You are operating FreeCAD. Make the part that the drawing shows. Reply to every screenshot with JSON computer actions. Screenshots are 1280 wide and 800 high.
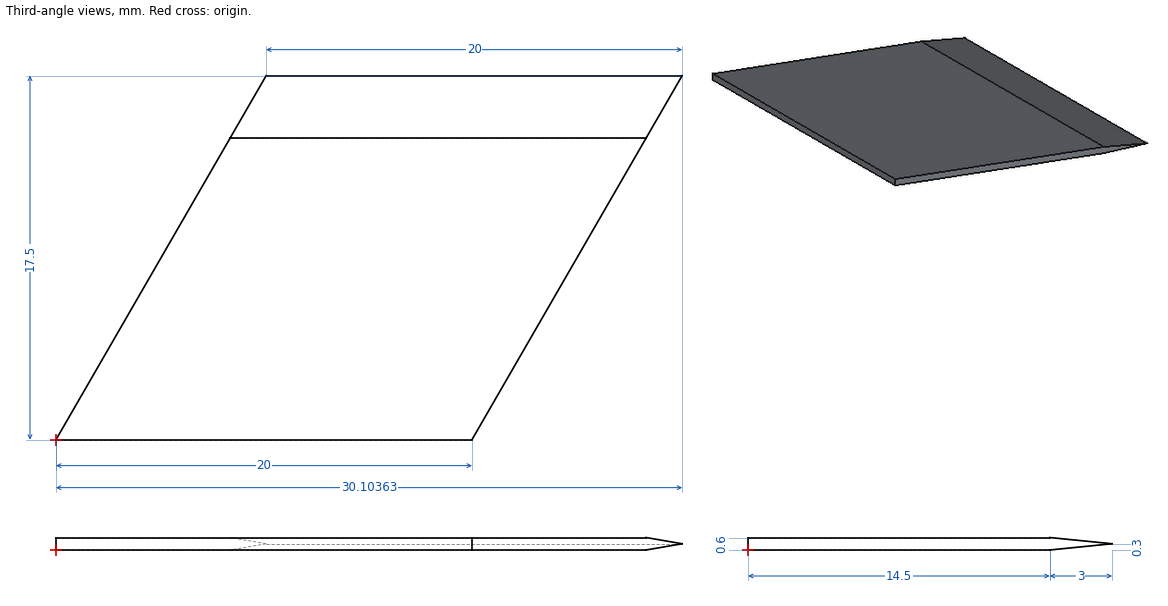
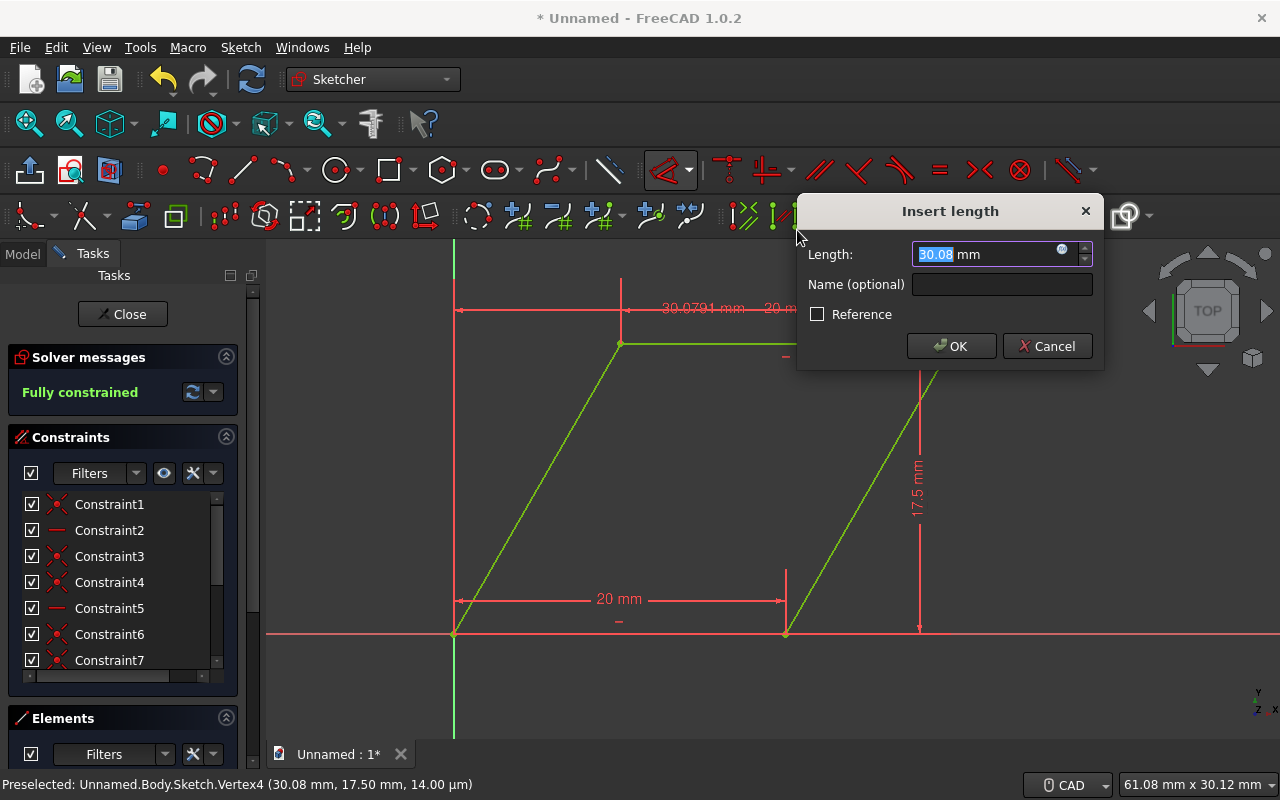
{"action": "type", "text": "30.10363"}
{"action": "key", "text": "Return"}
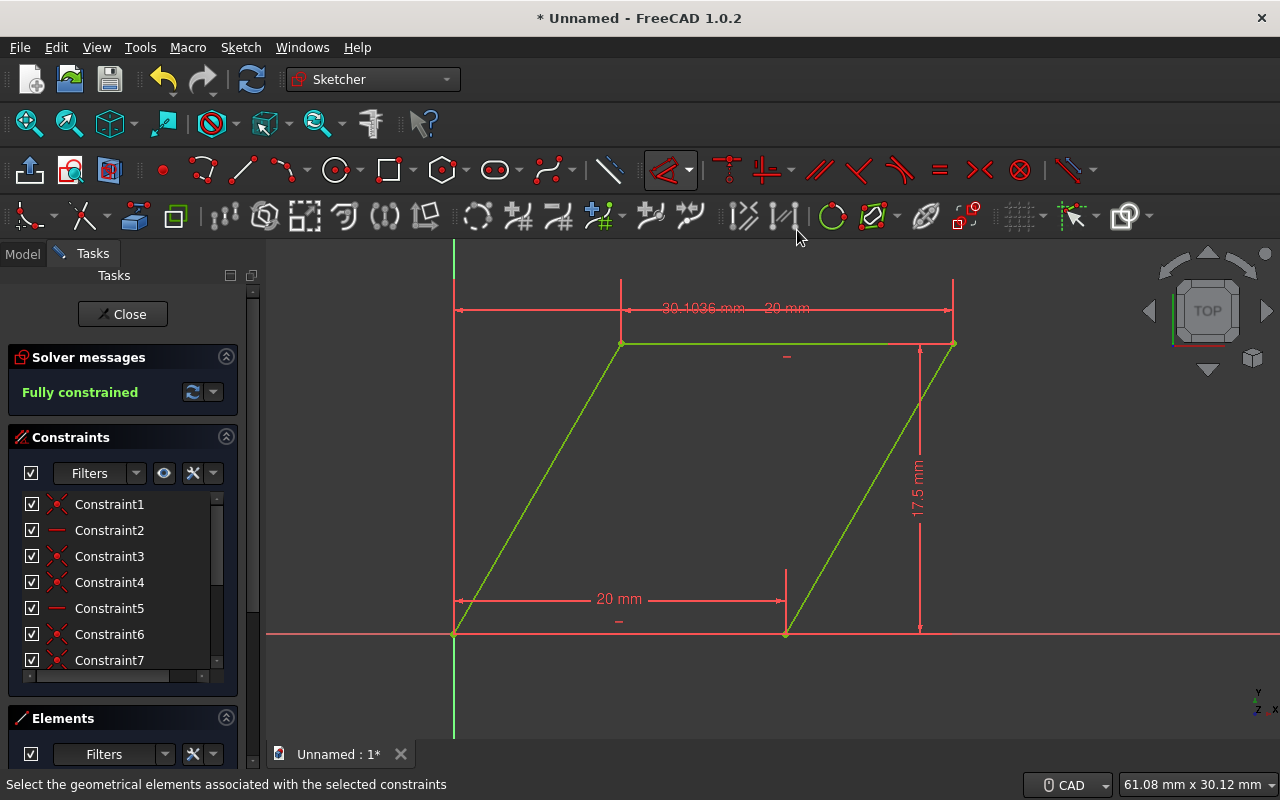
{"action": "left_click", "coordinate": [123, 314]}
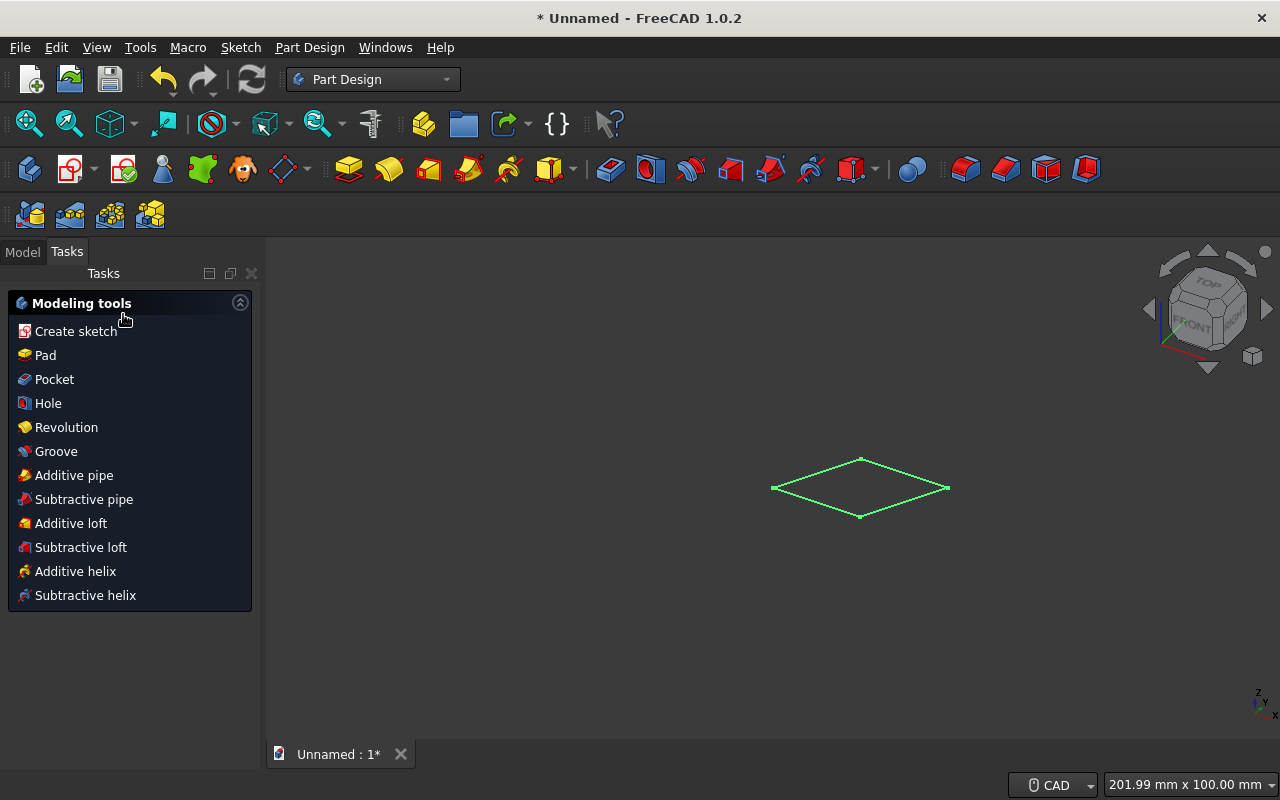
{"action": "left_click", "coordinate": [350, 170]}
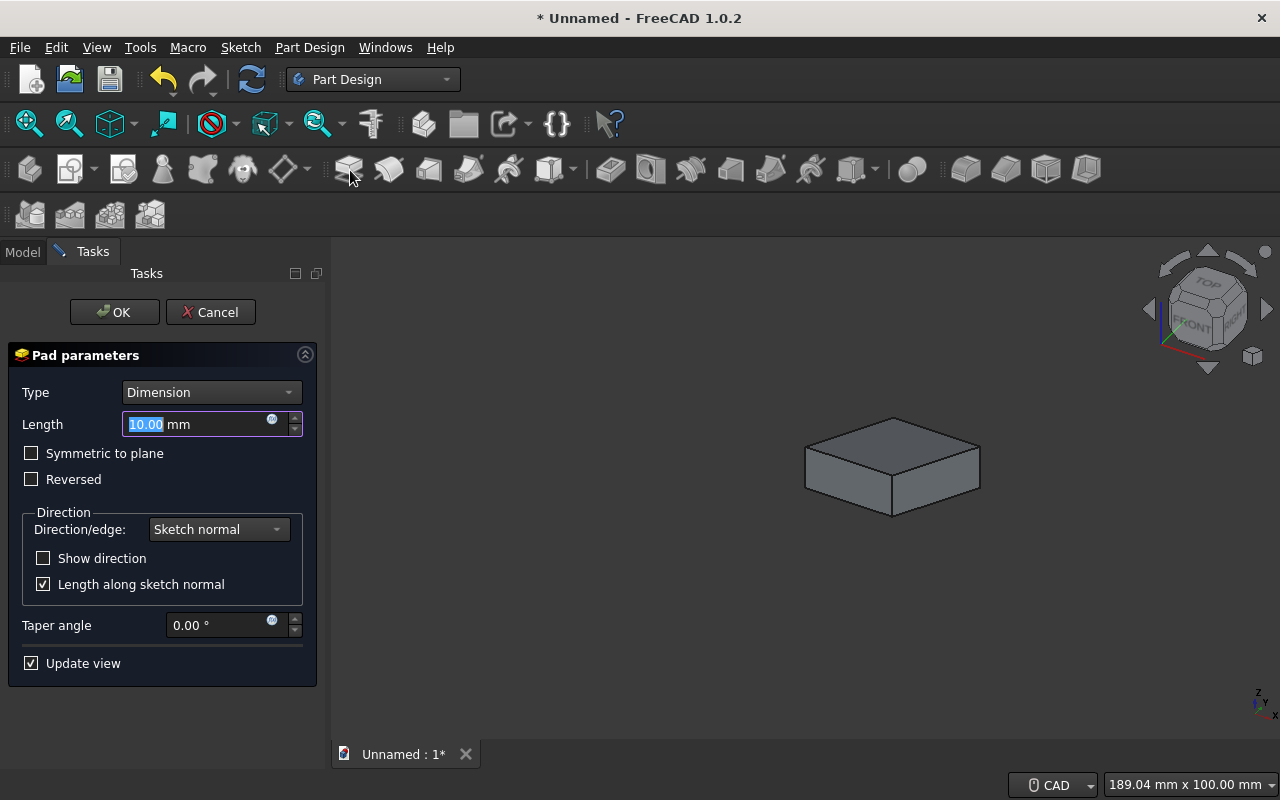
{"action": "type", "text": "0.6"}
{"action": "key", "text": "Tab"}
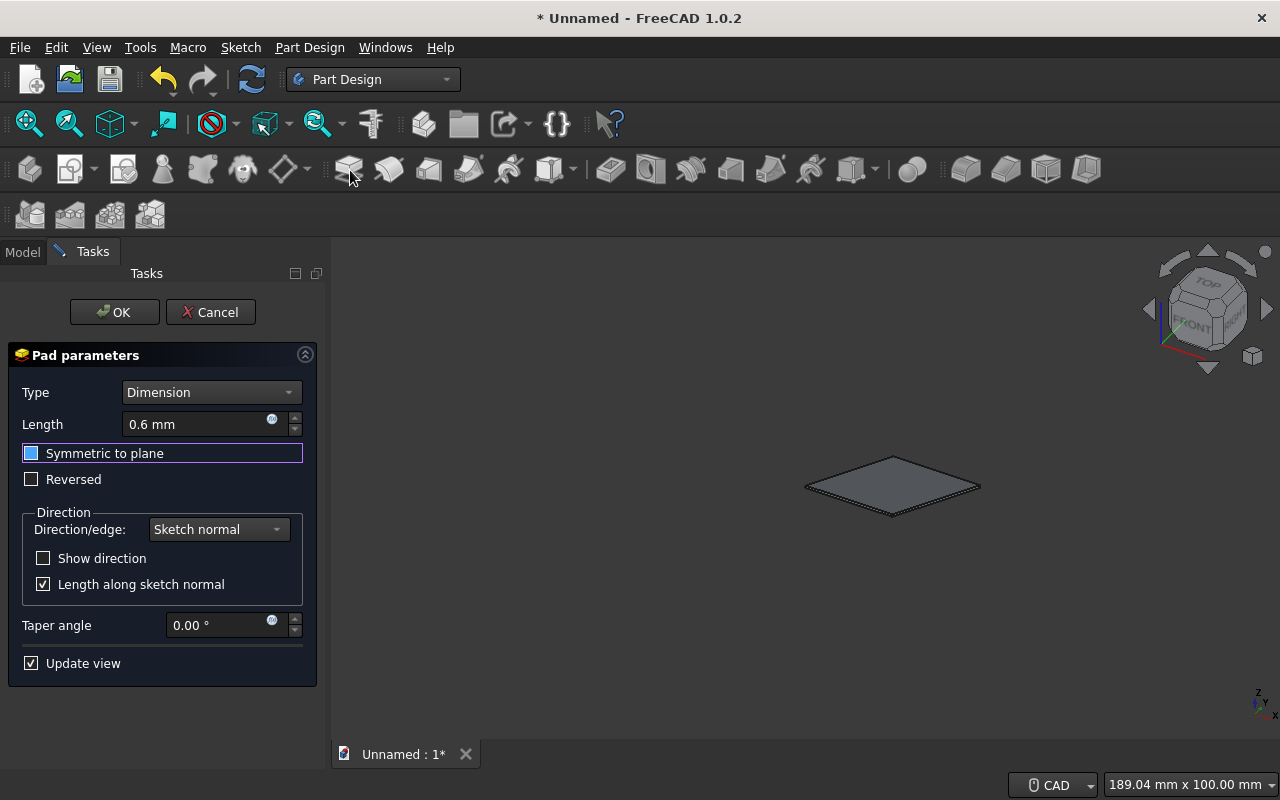
{"action": "left_click", "coordinate": [115, 312]}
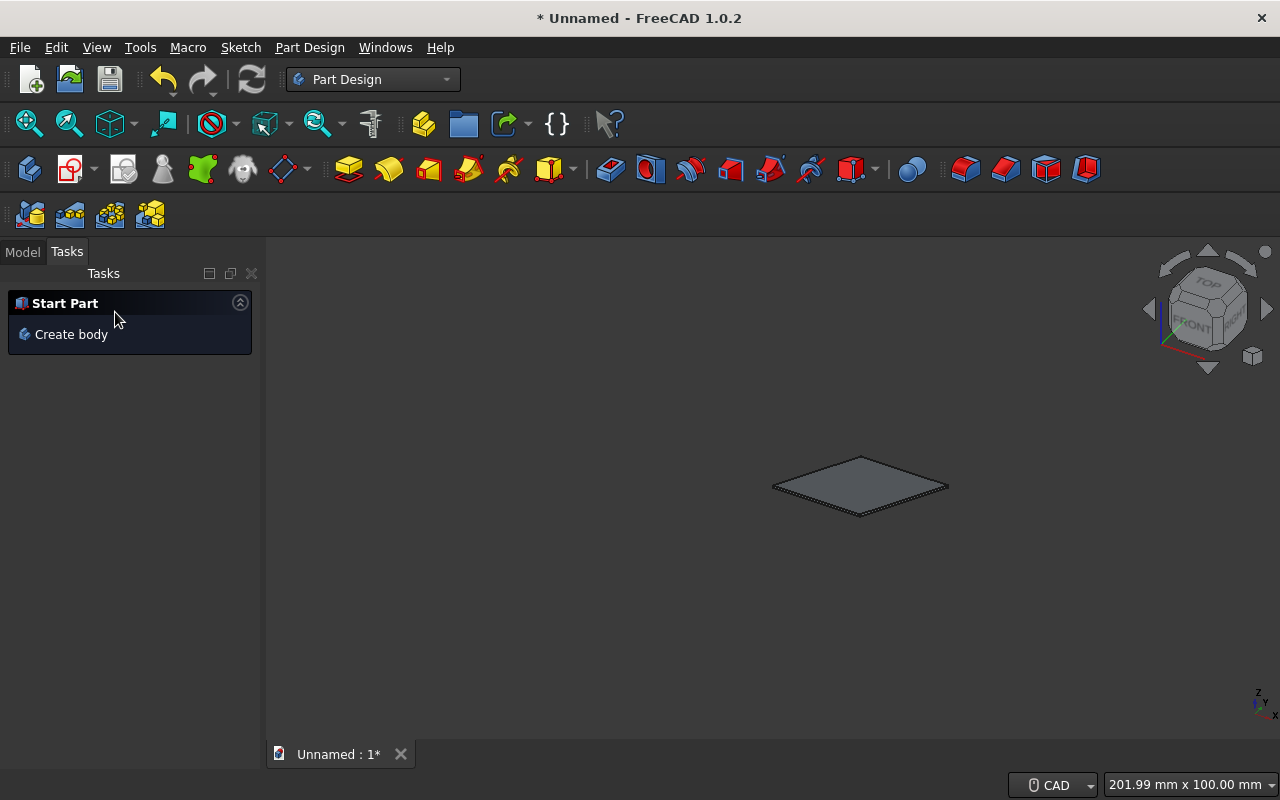
{"action": "left_click", "coordinate": [30, 124]}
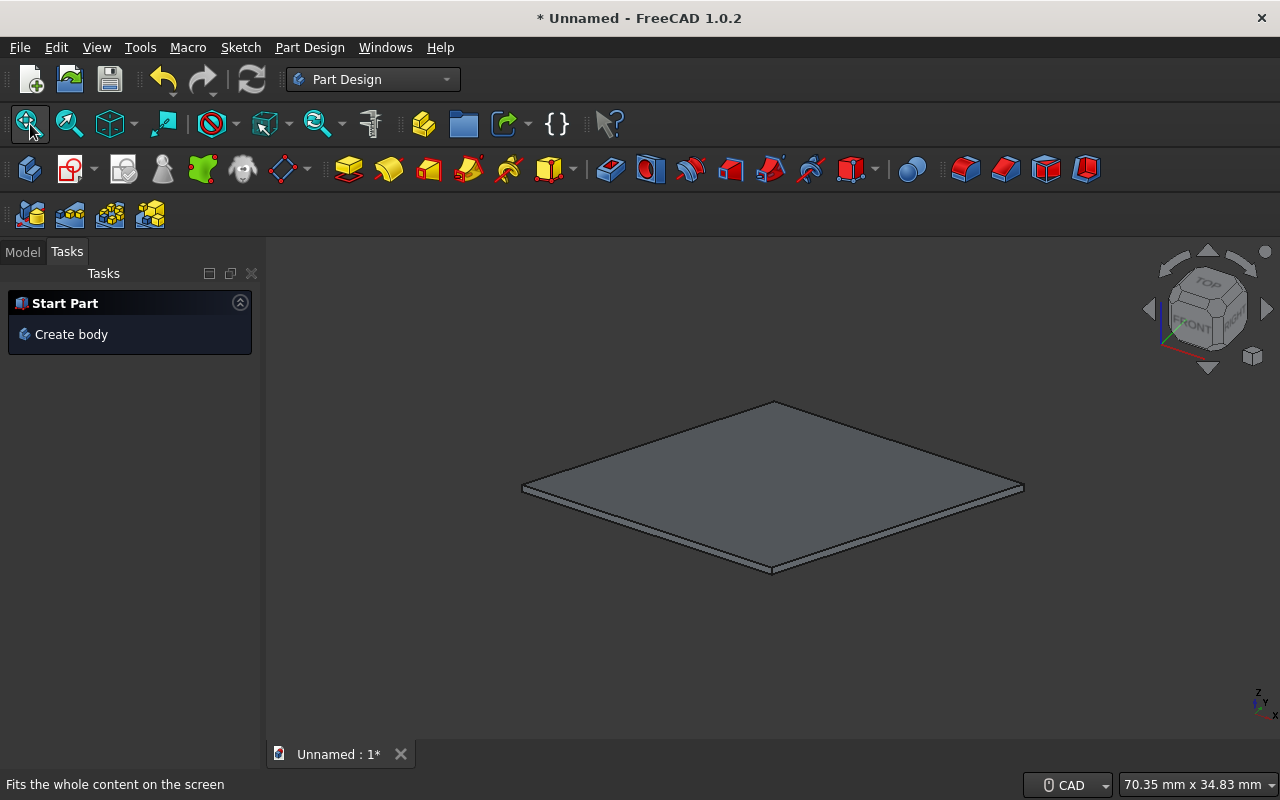
{"action": "left_click", "coordinate": [70, 170]}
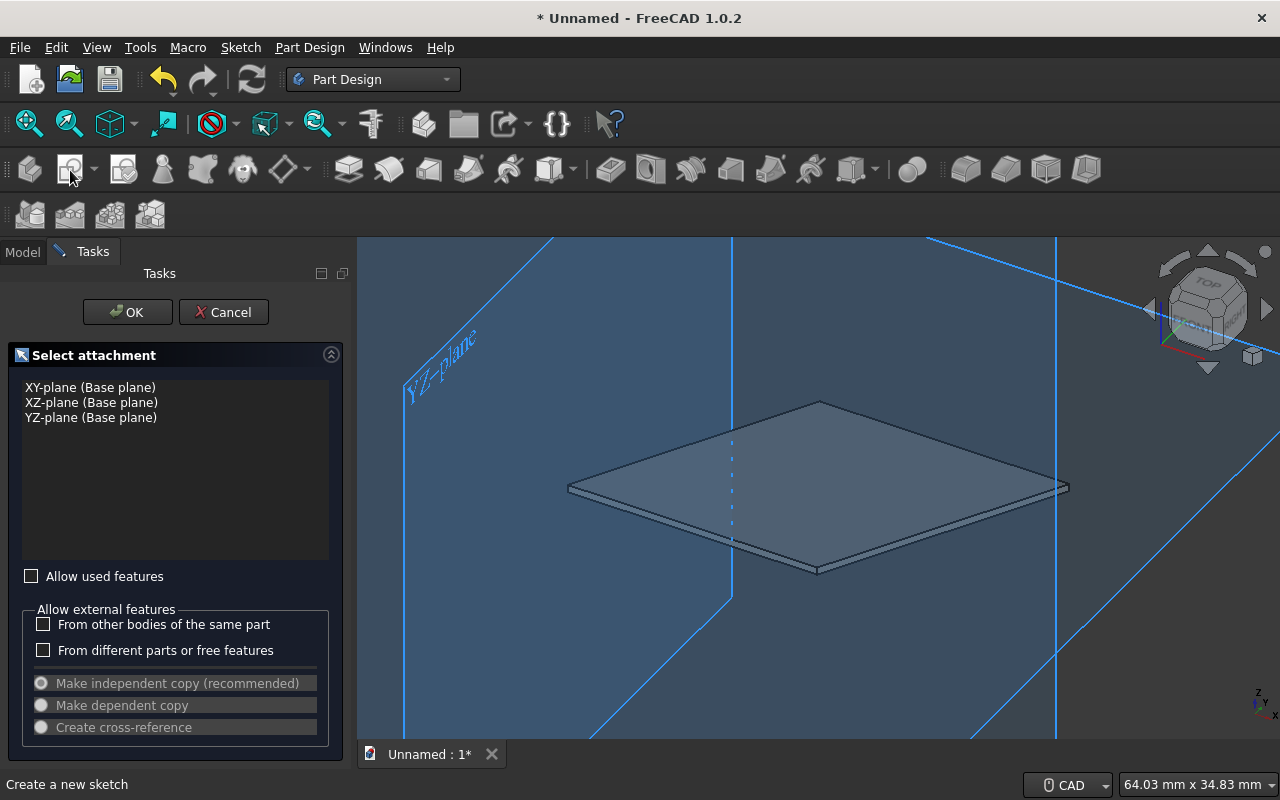
{"action": "left_click", "coordinate": [82, 418]}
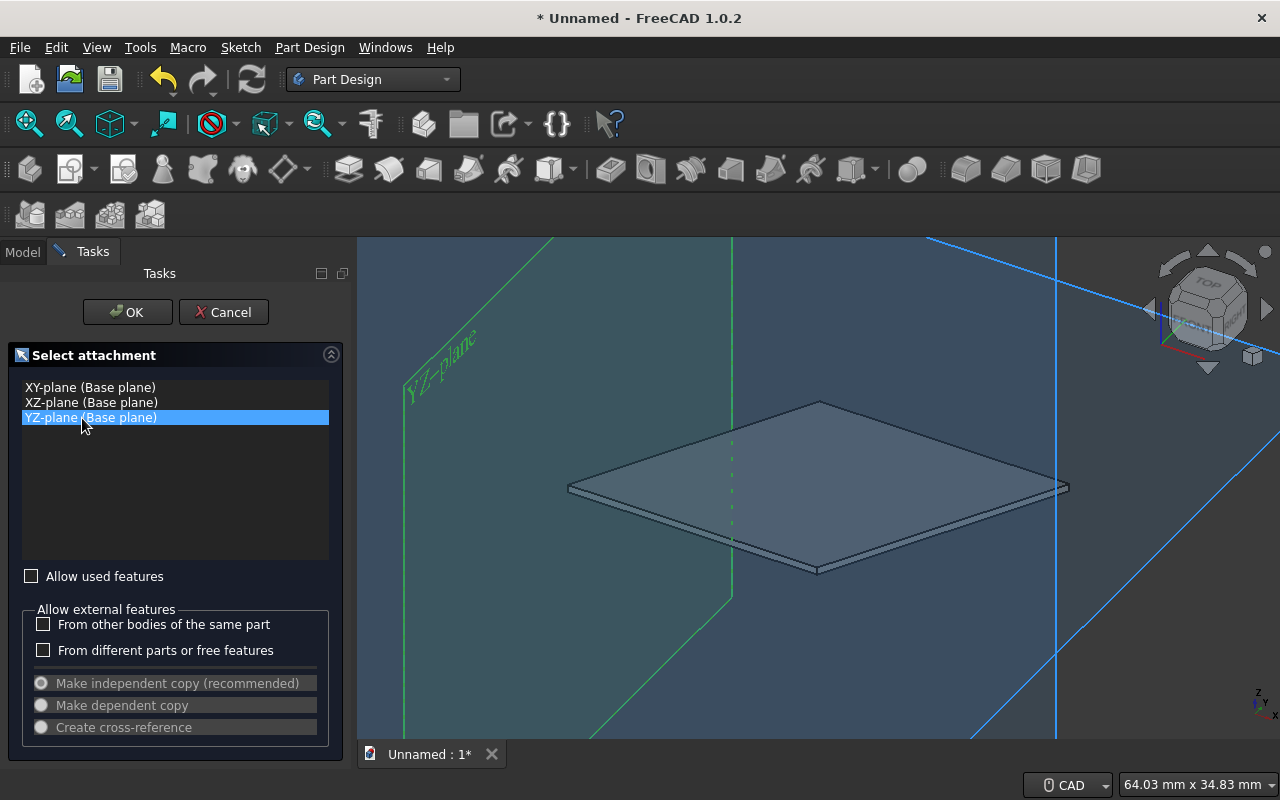
{"action": "left_click", "coordinate": [128, 312]}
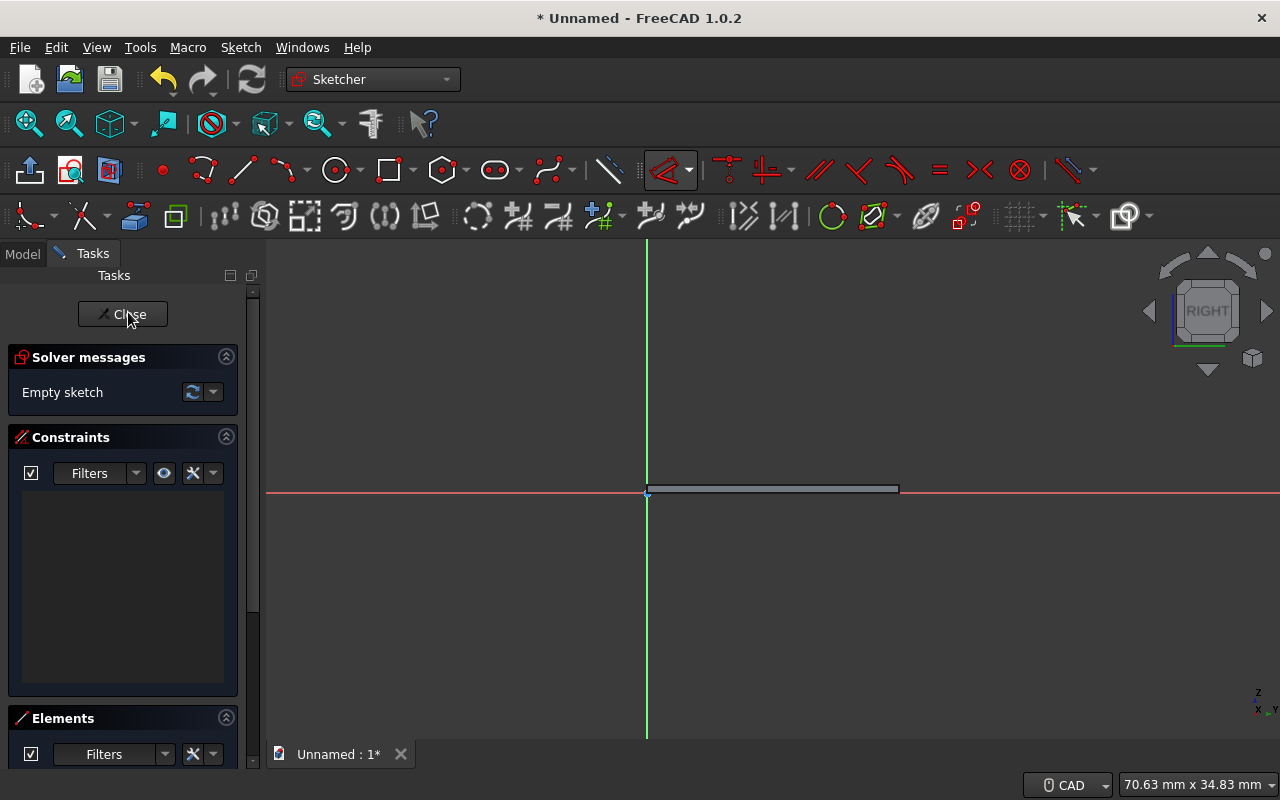
{"action": "left_click", "coordinate": [110, 170]}